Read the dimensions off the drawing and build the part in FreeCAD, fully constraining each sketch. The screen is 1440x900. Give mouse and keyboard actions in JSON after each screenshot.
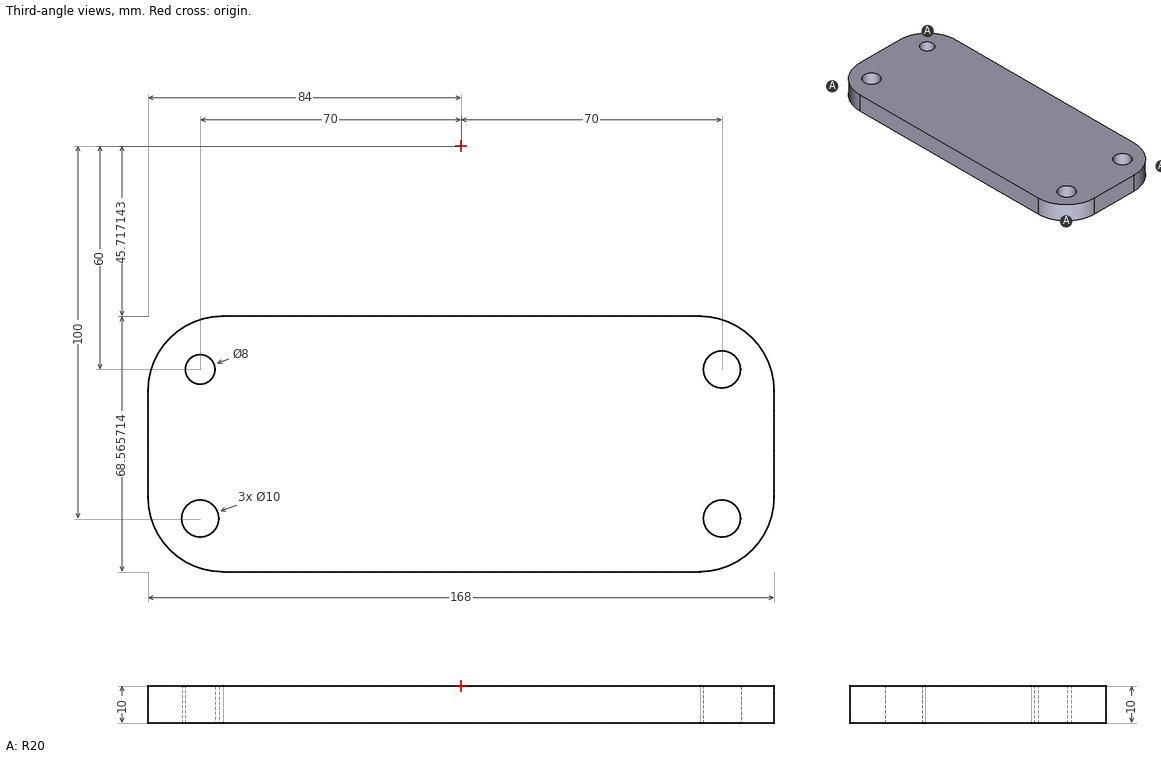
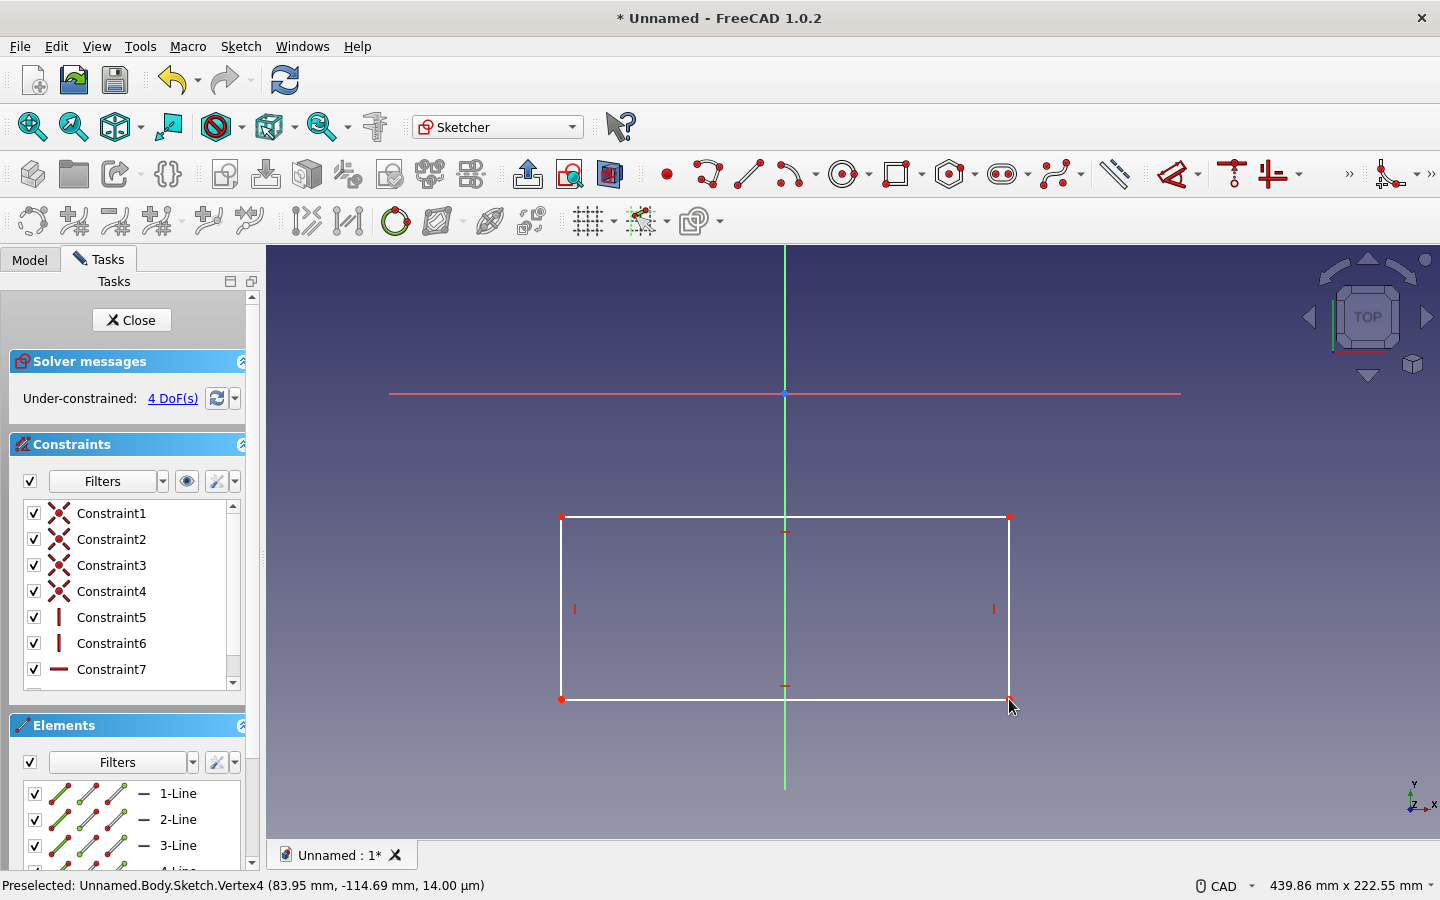
{"action": "left_click", "coordinate": [695, 700]}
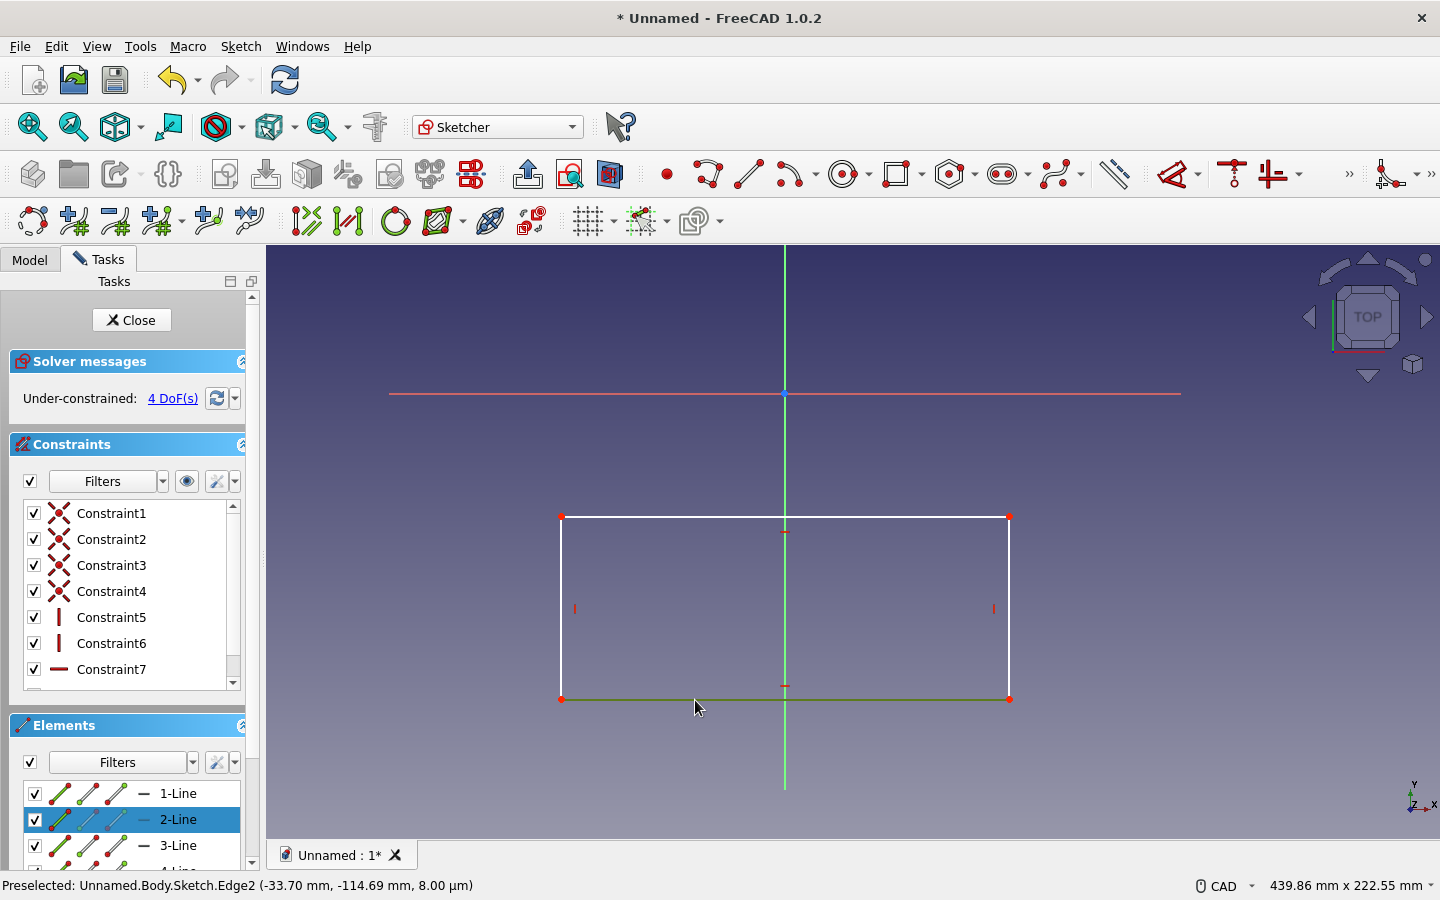
{"action": "key", "text": "l"}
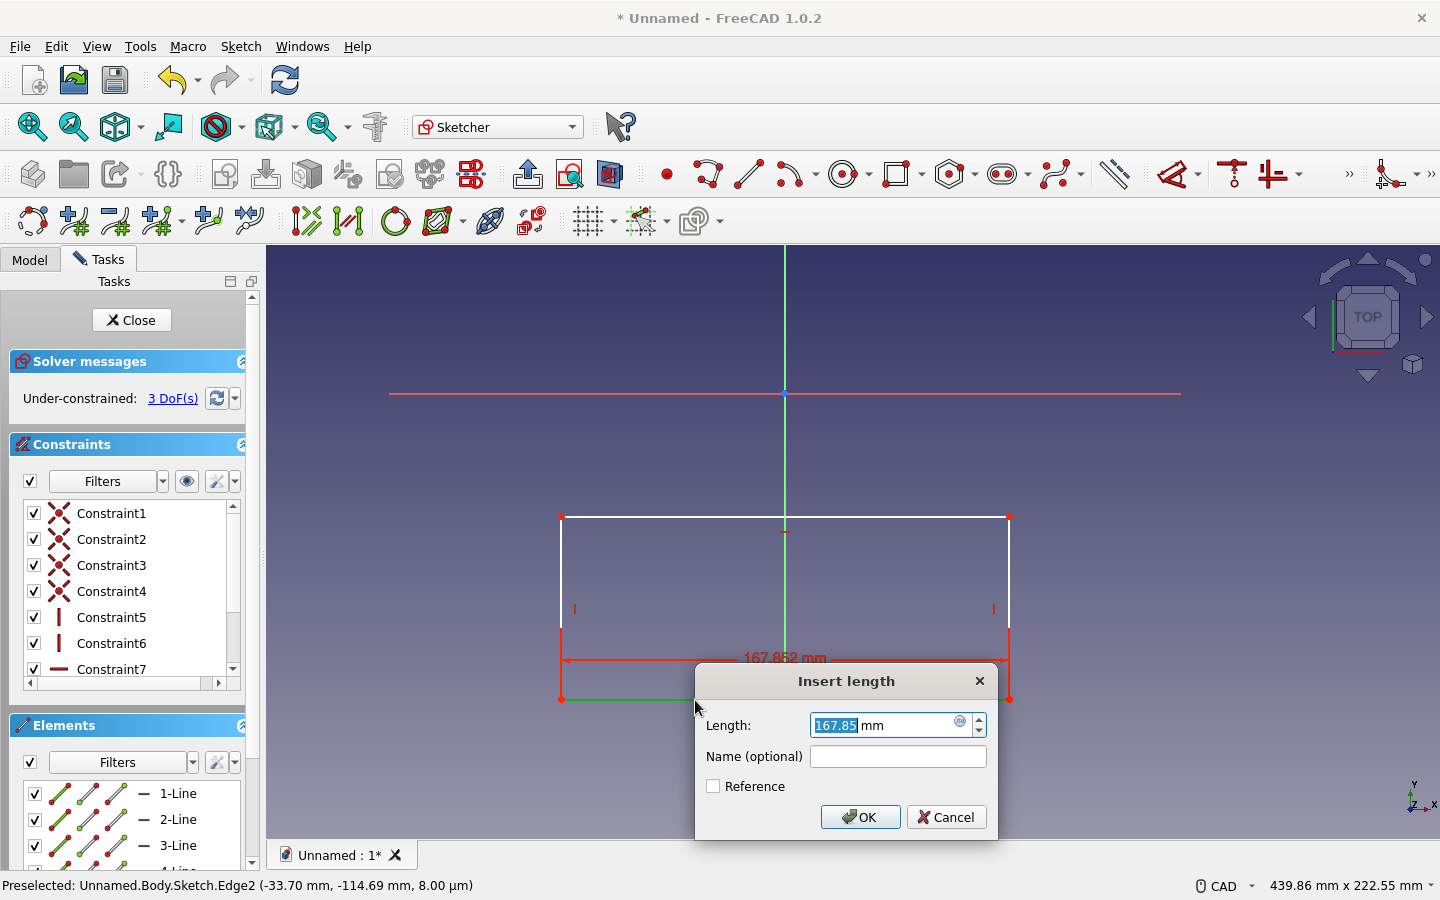
{"action": "type", "text": "168"}
{"action": "key", "text": "Return"}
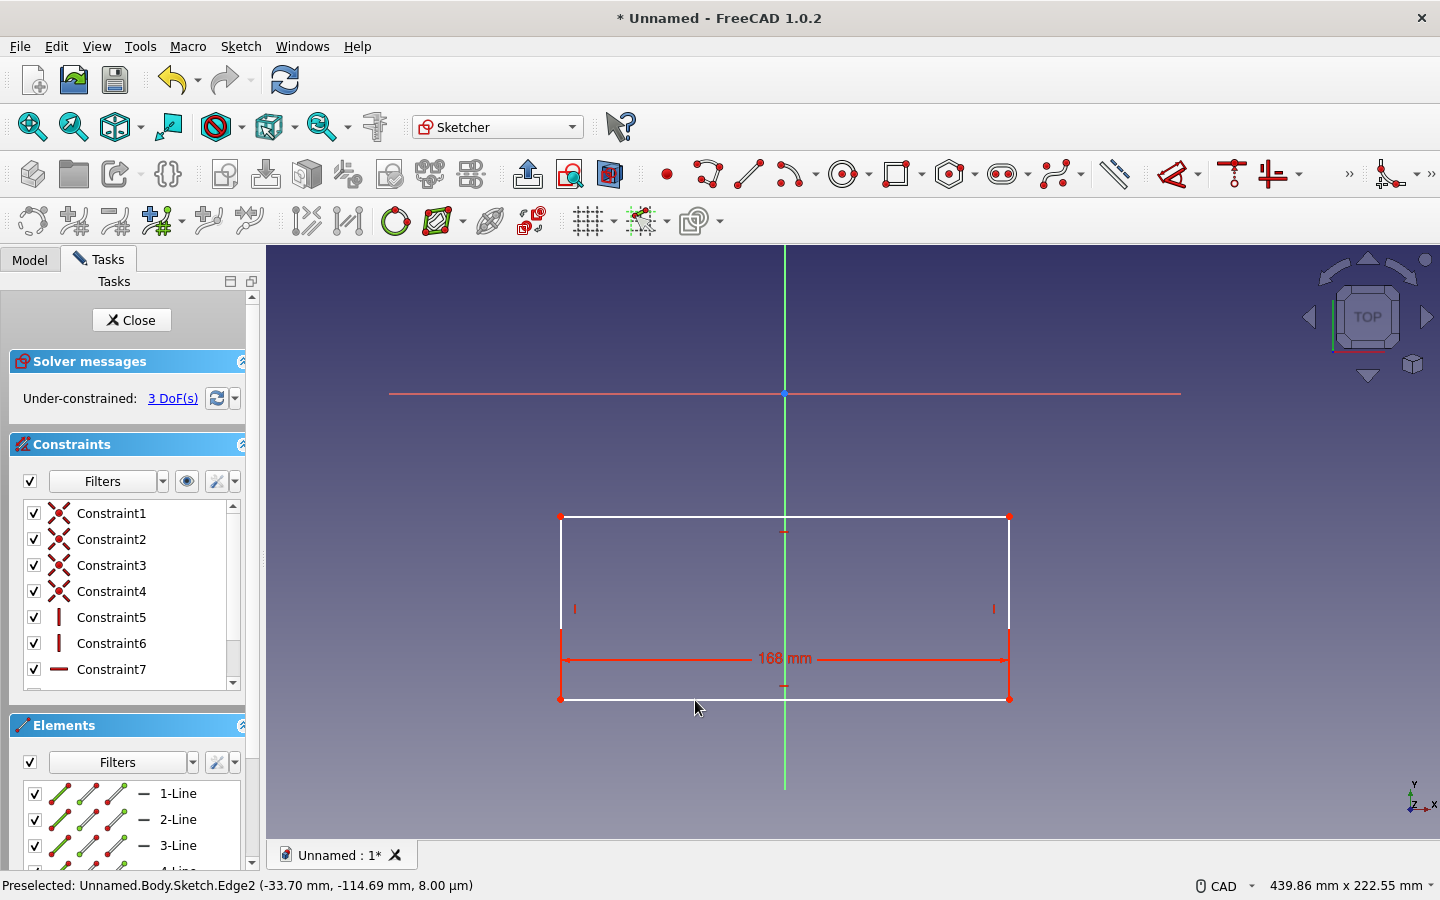
{"action": "left_click", "coordinate": [561, 517]}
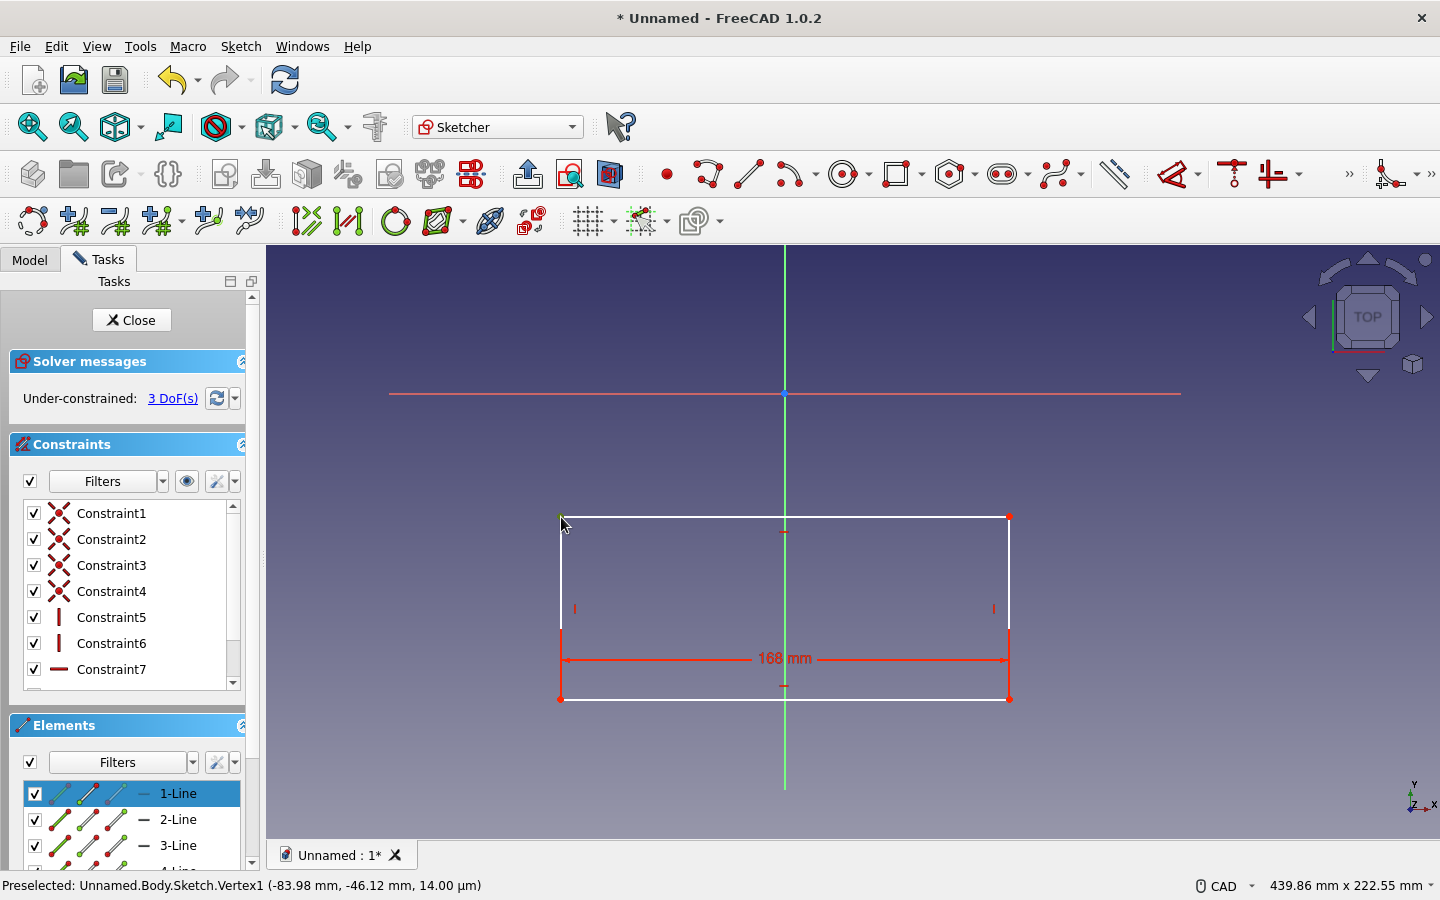
{"action": "key", "text": "l"}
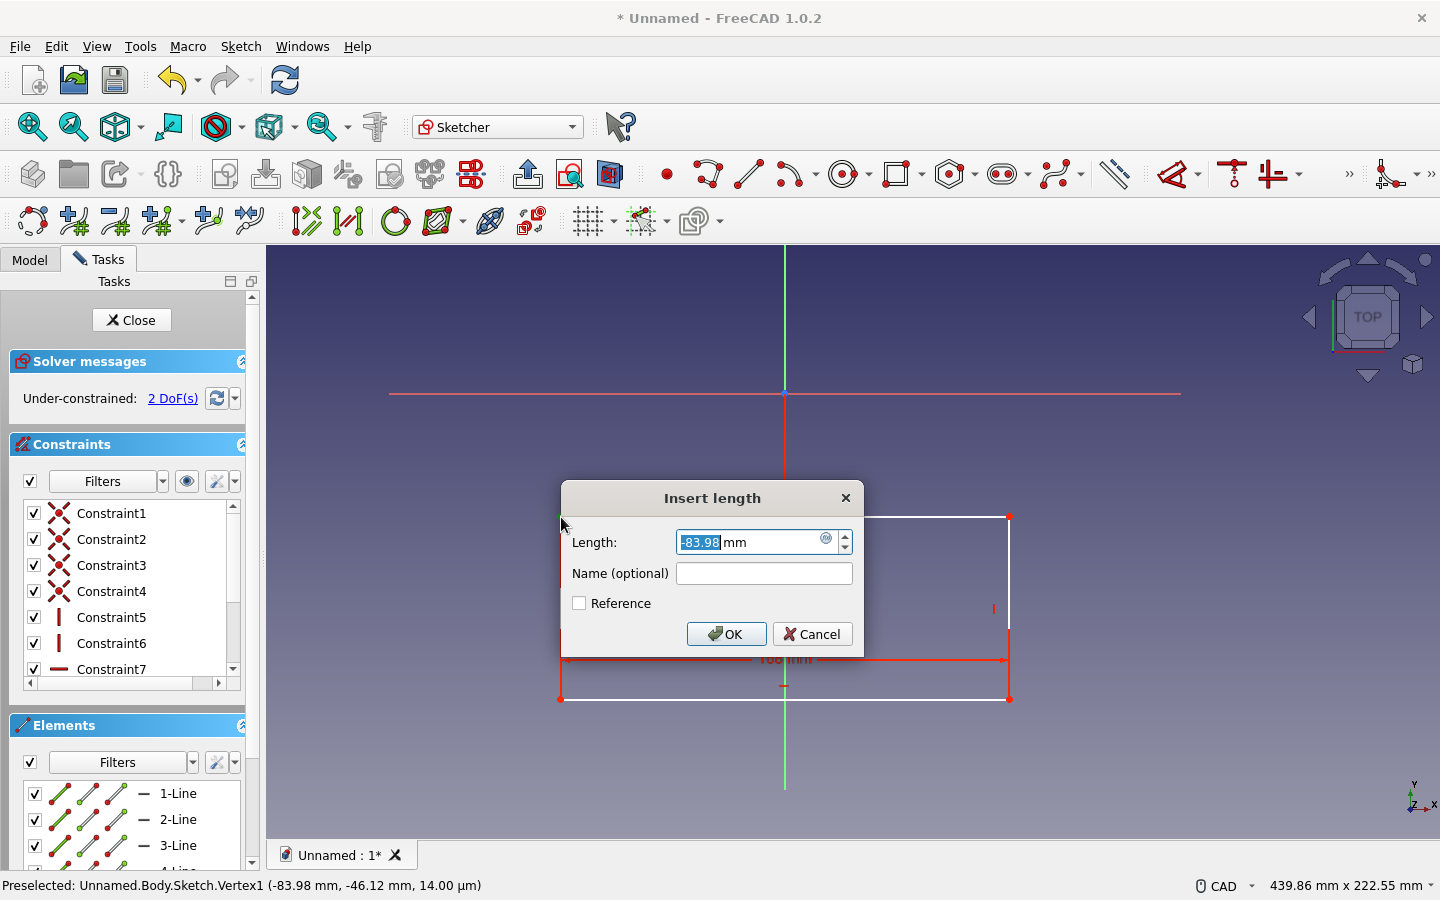
{"action": "type", "text": "-84"}
{"action": "key", "text": "Return"}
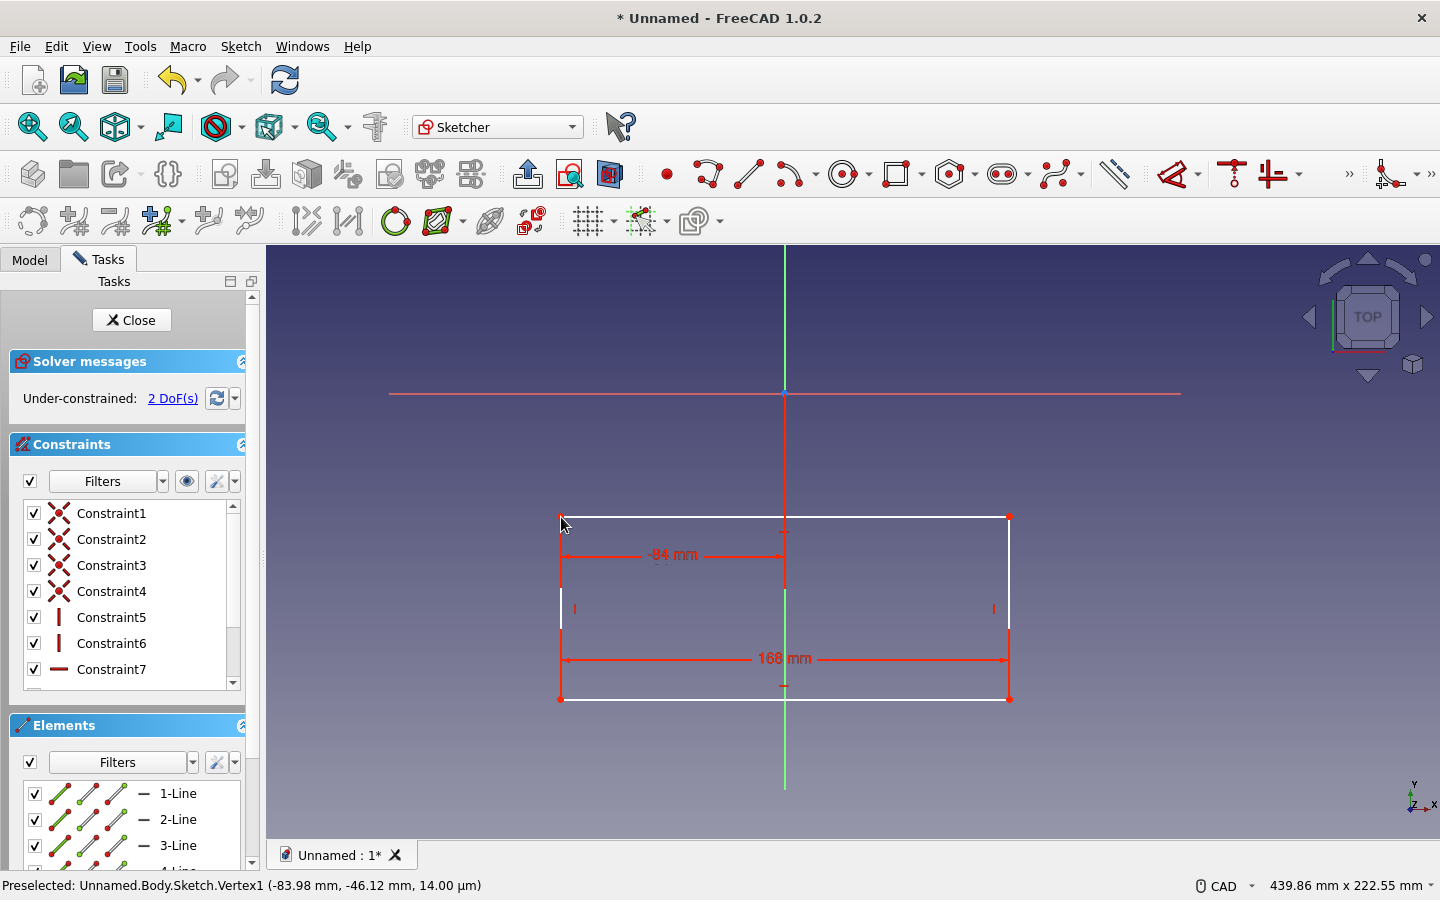
{"action": "left_click", "coordinate": [561, 572]}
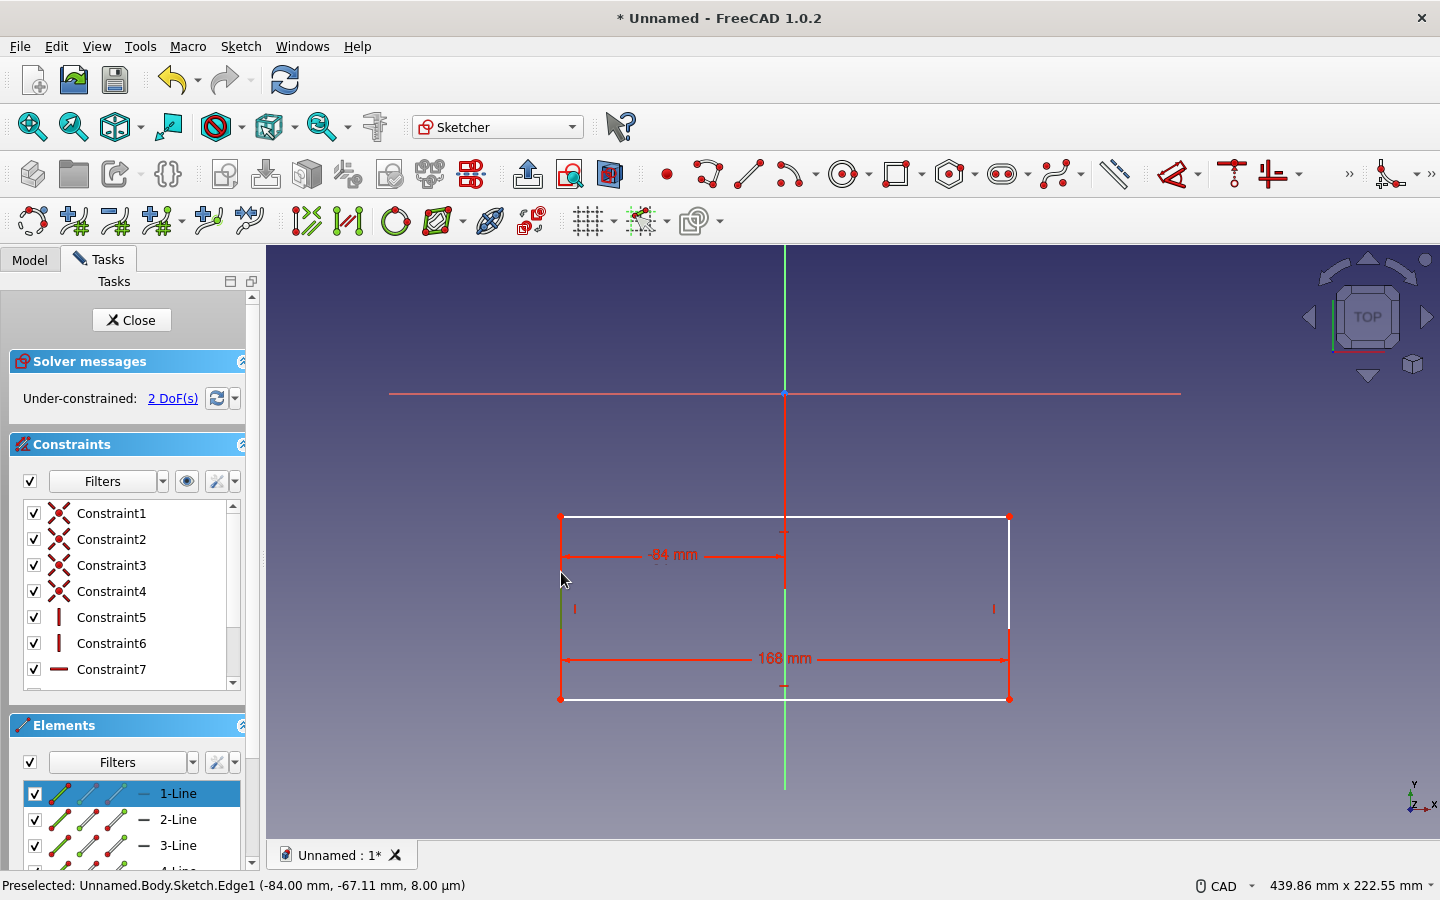
{"action": "key", "text": "i"}